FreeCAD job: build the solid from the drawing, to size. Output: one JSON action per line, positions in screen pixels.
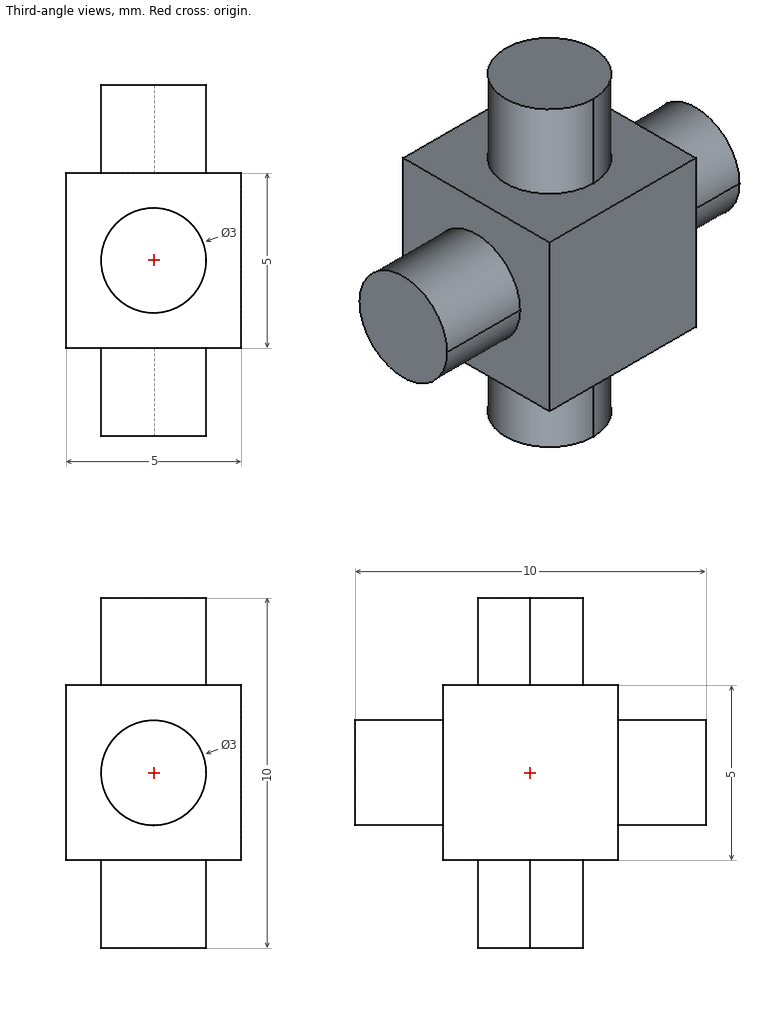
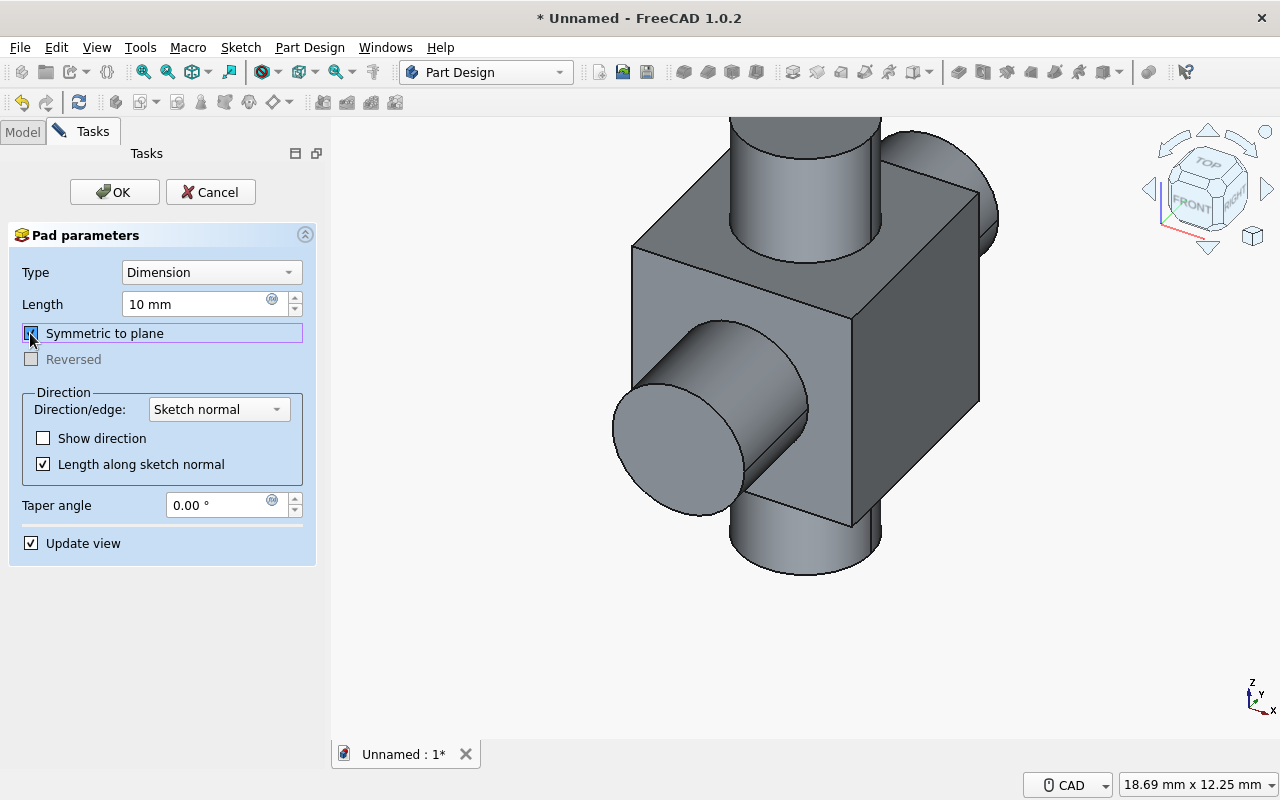
{"action": "left_click", "coordinate": [115, 192]}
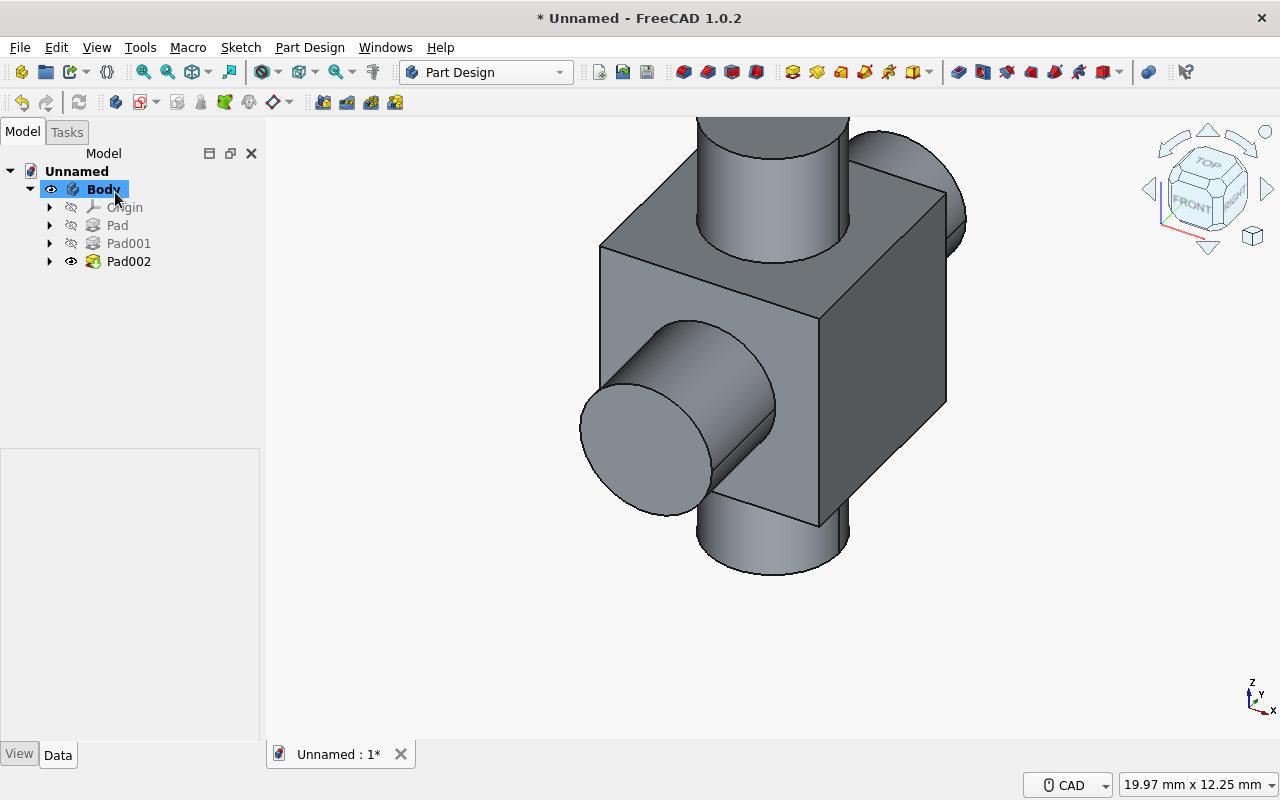
{"action": "key", "text": "0"}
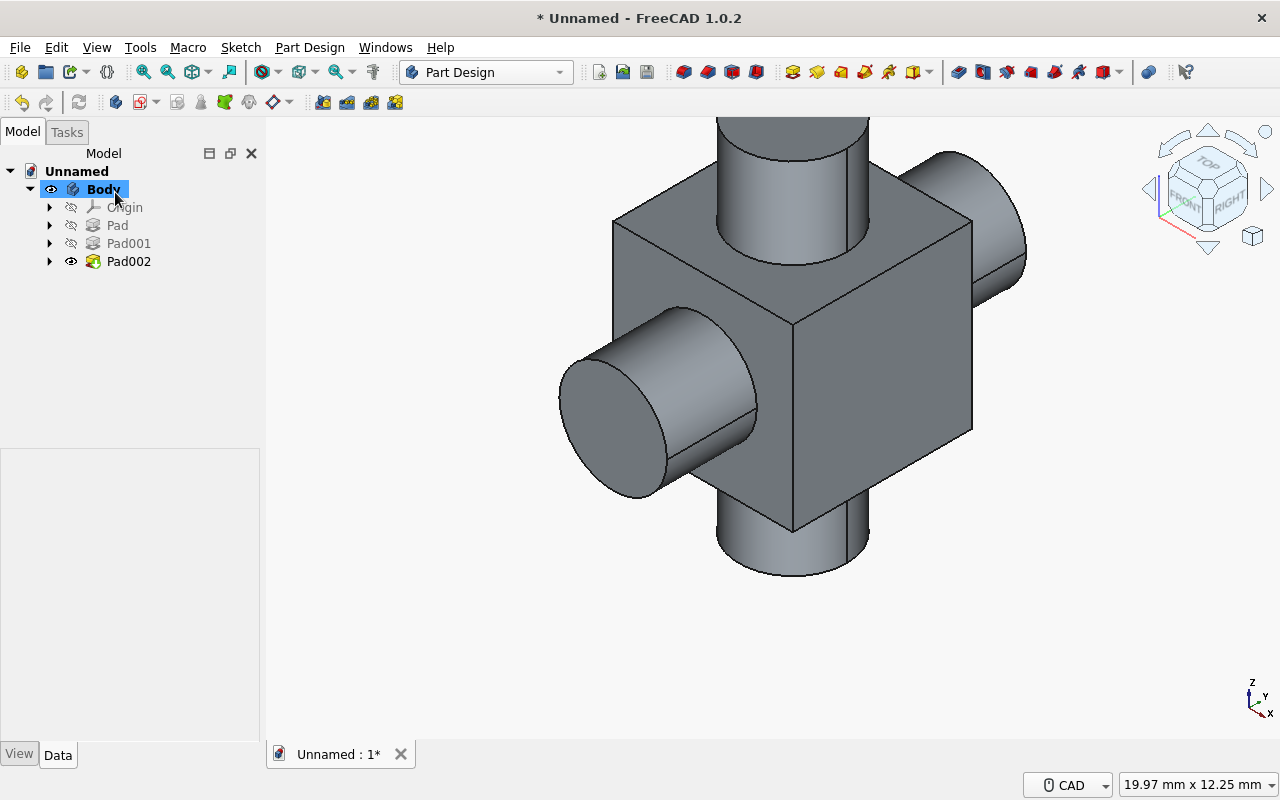
{"action": "left_click", "coordinate": [144, 72]}